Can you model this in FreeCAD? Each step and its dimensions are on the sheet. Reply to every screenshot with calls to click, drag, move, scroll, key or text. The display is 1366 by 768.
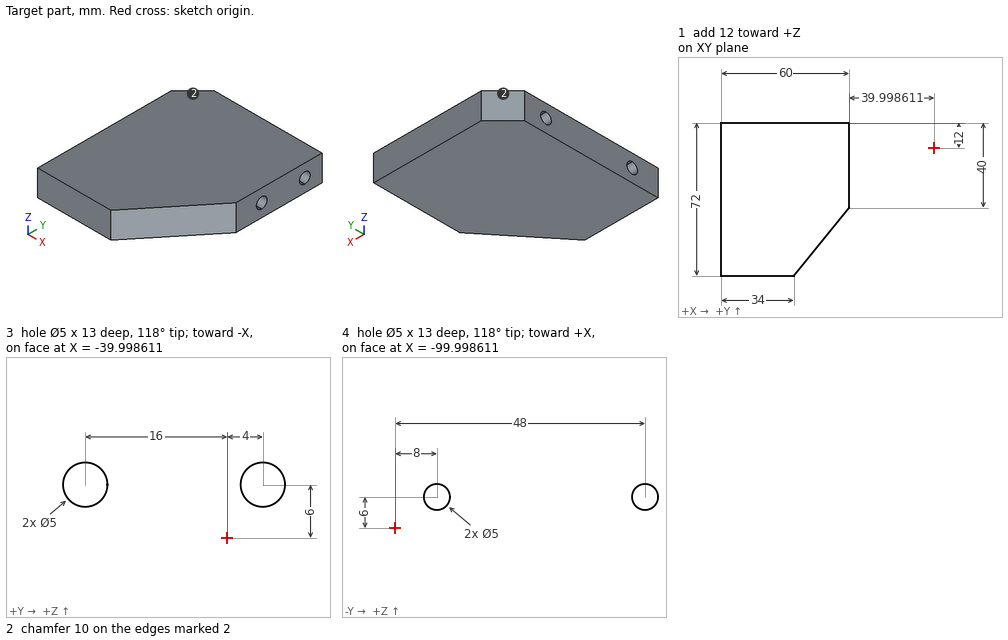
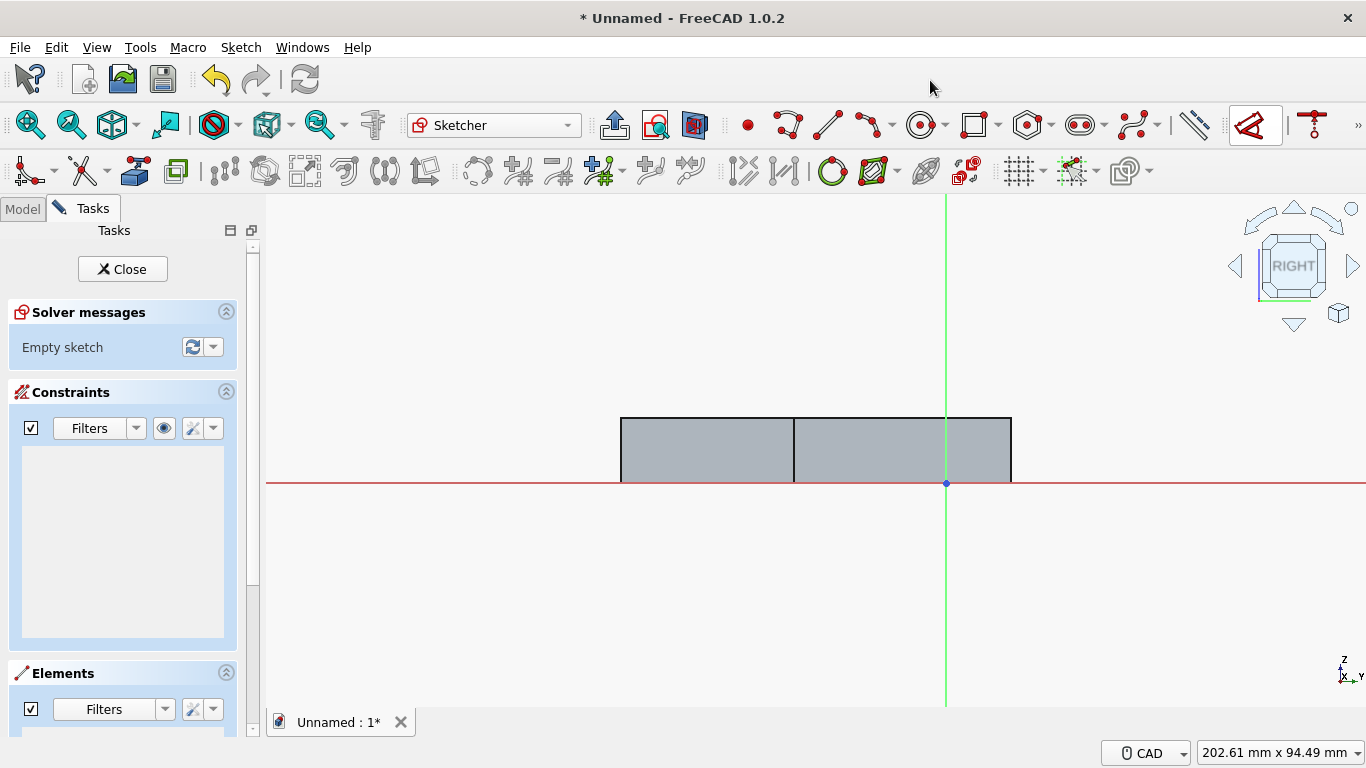
scroll(956, 462, up, 8)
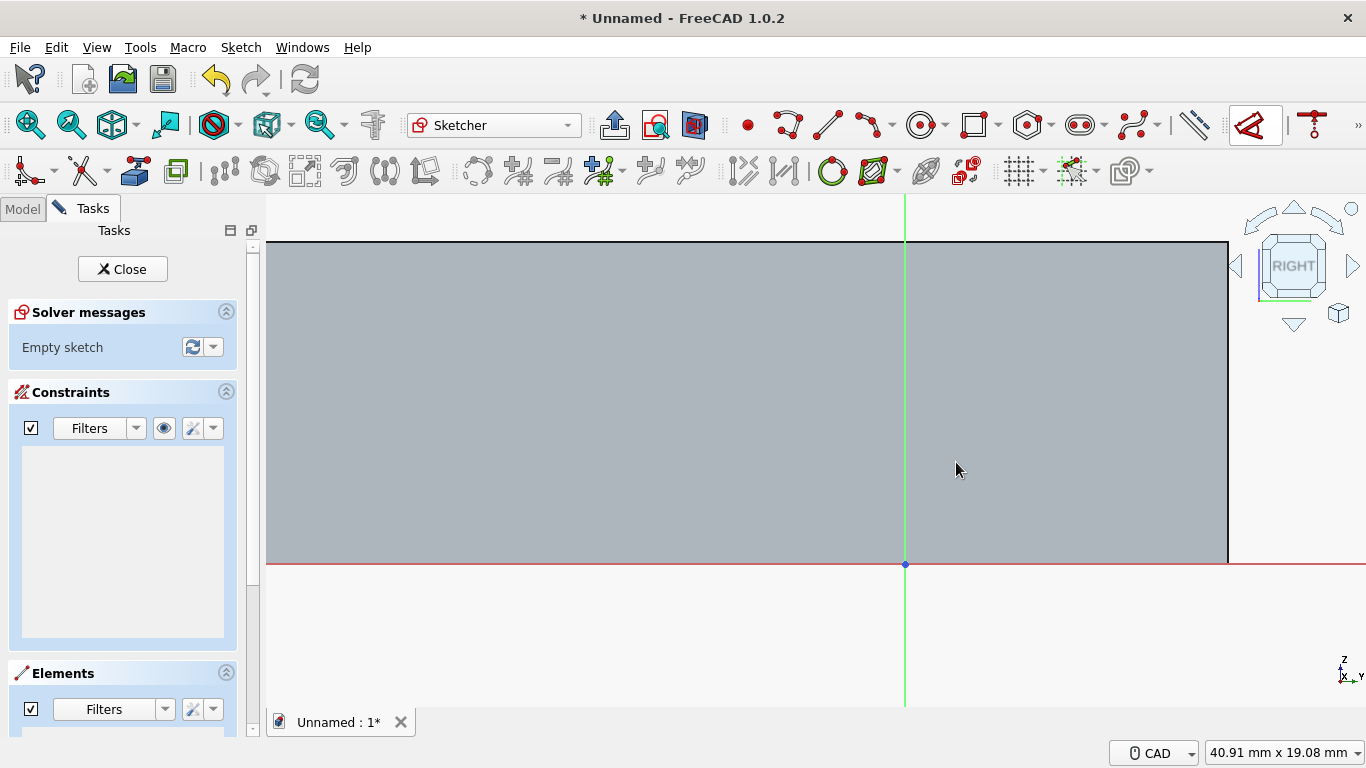
click(922, 126)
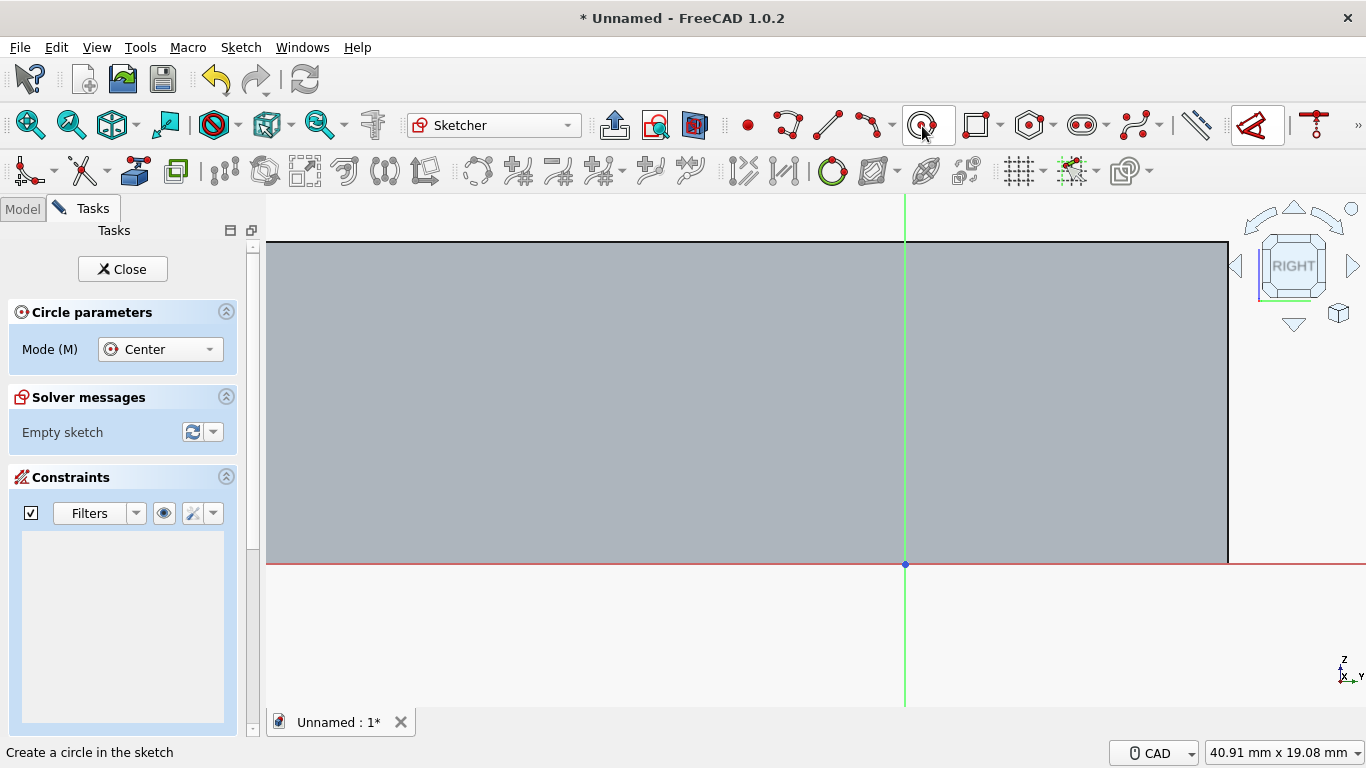
click(1013, 403)
move(1061, 355)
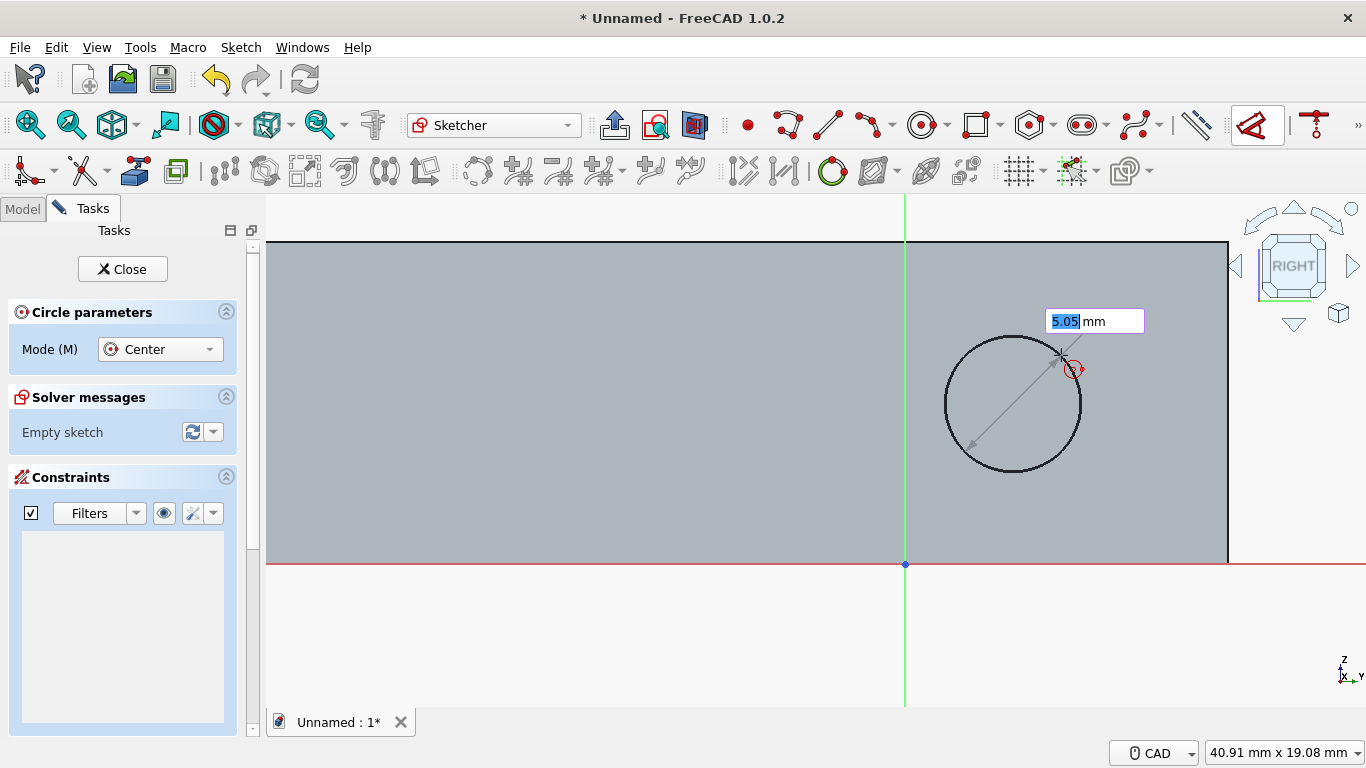
text(5)
key(Return)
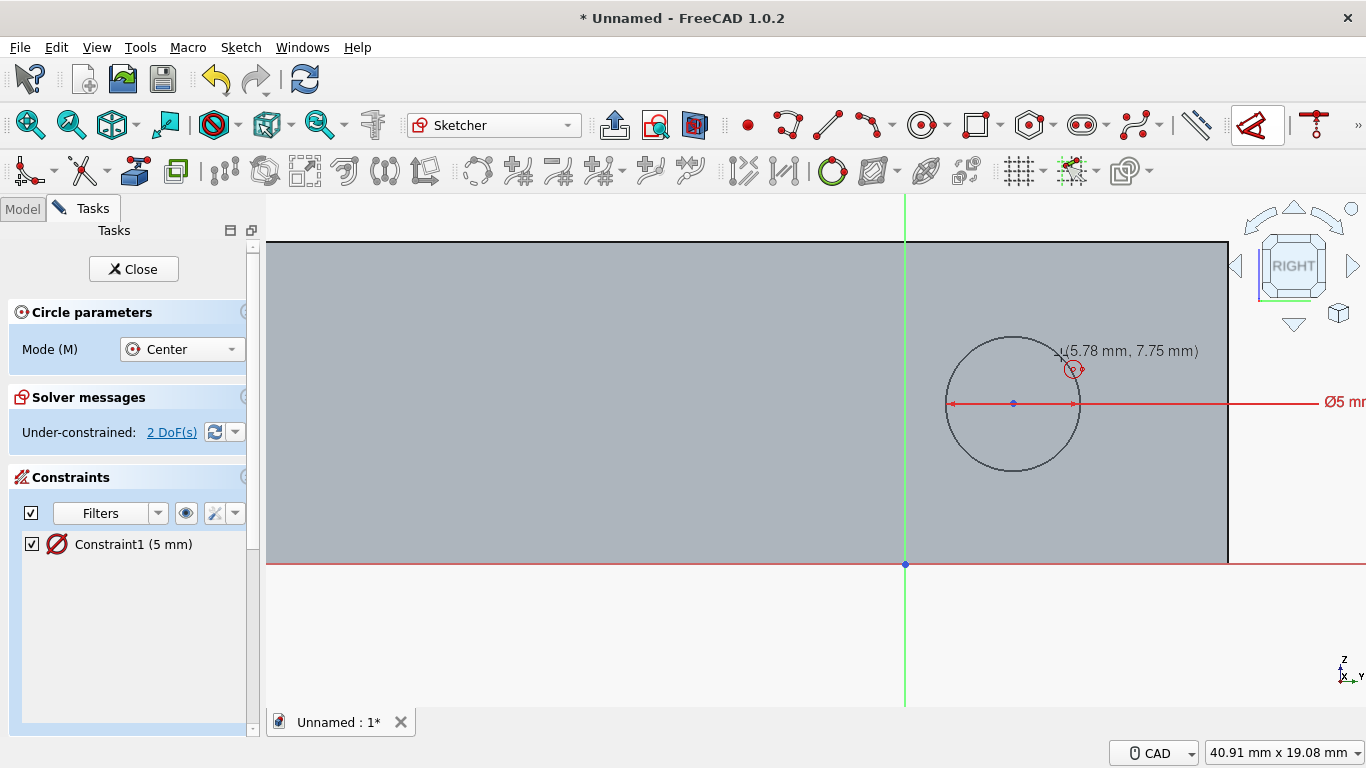
click(475, 403)
move(523, 355)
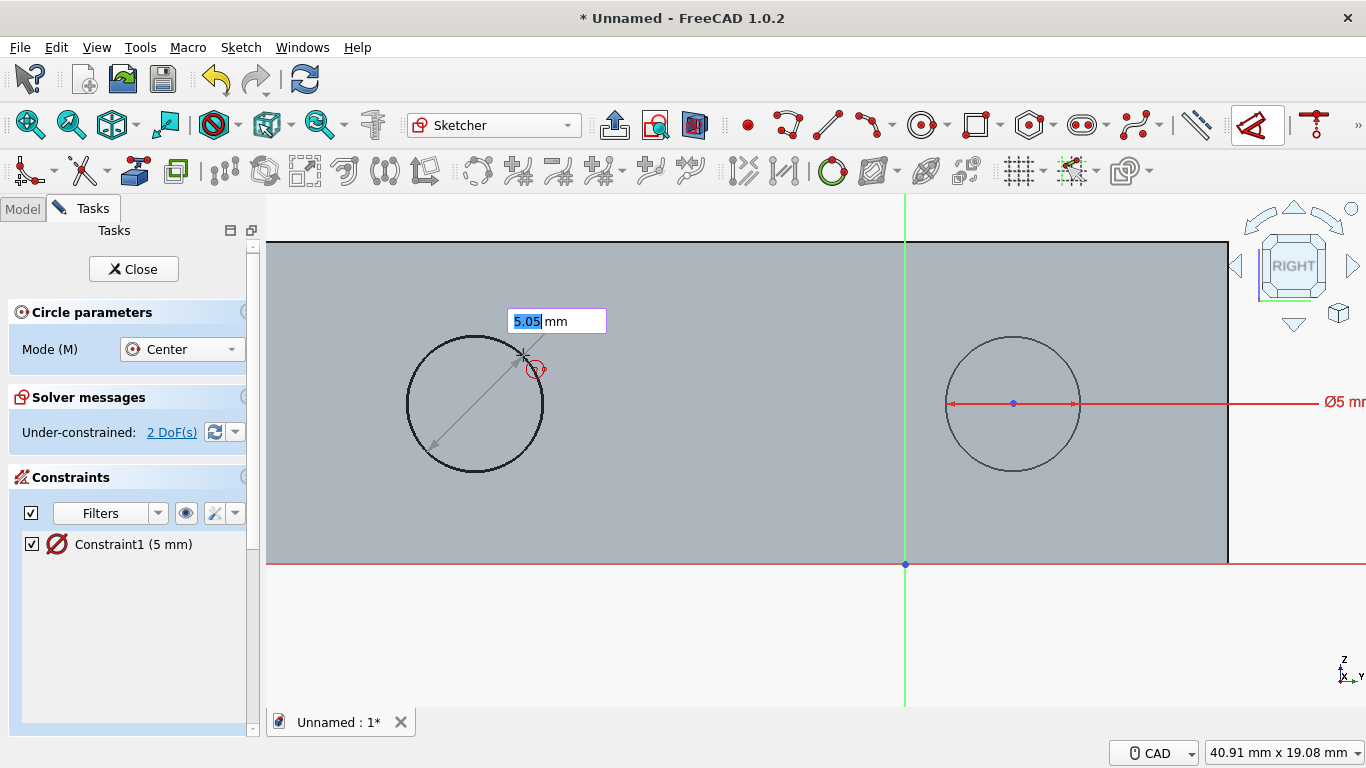
text(5)
key(Return)
key(Escape)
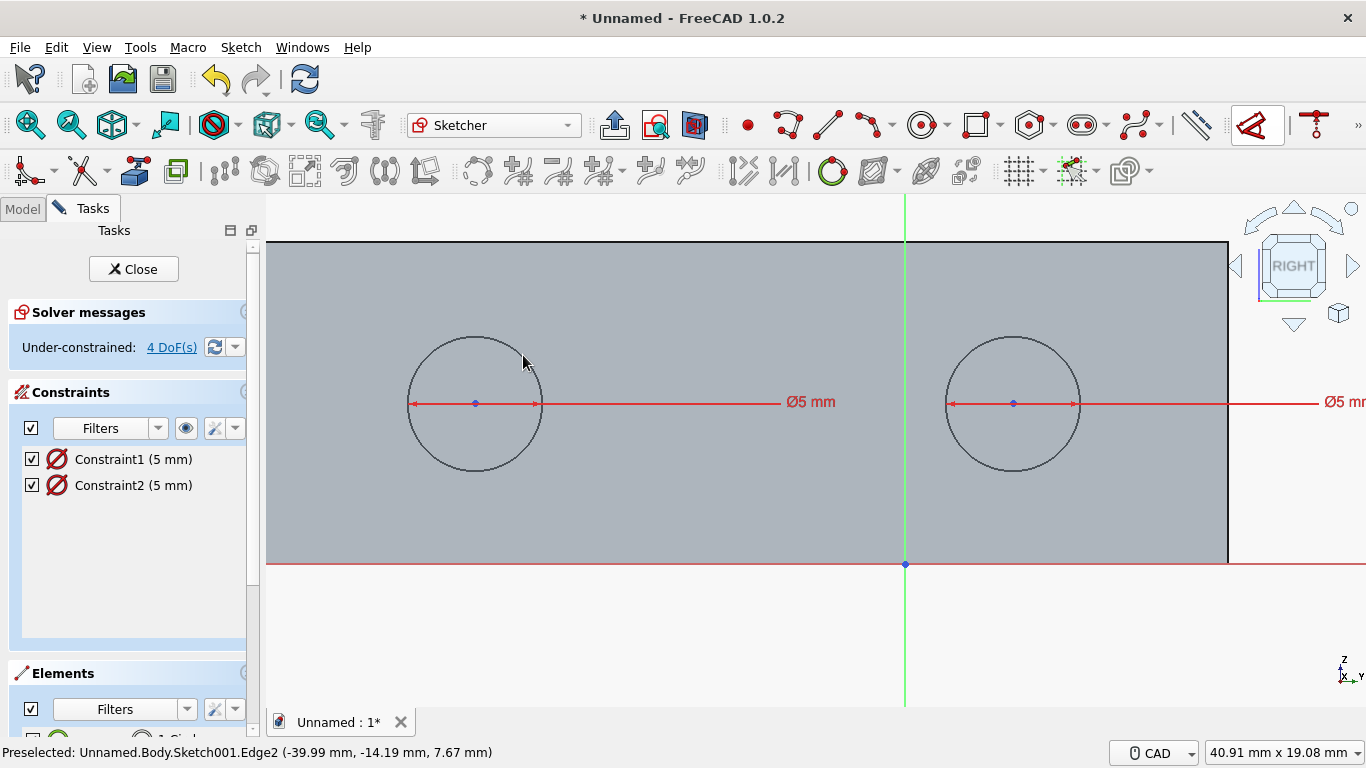
click(1013, 404)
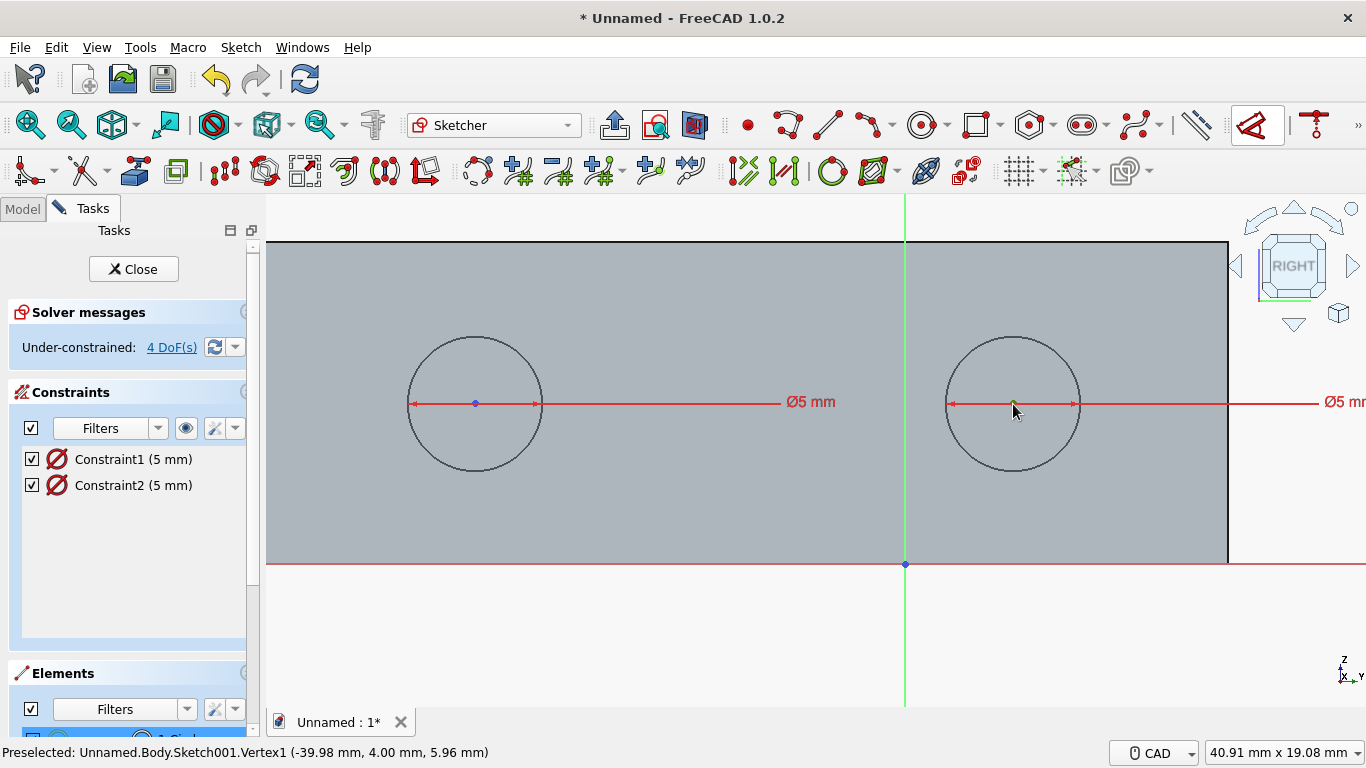
click(475, 404)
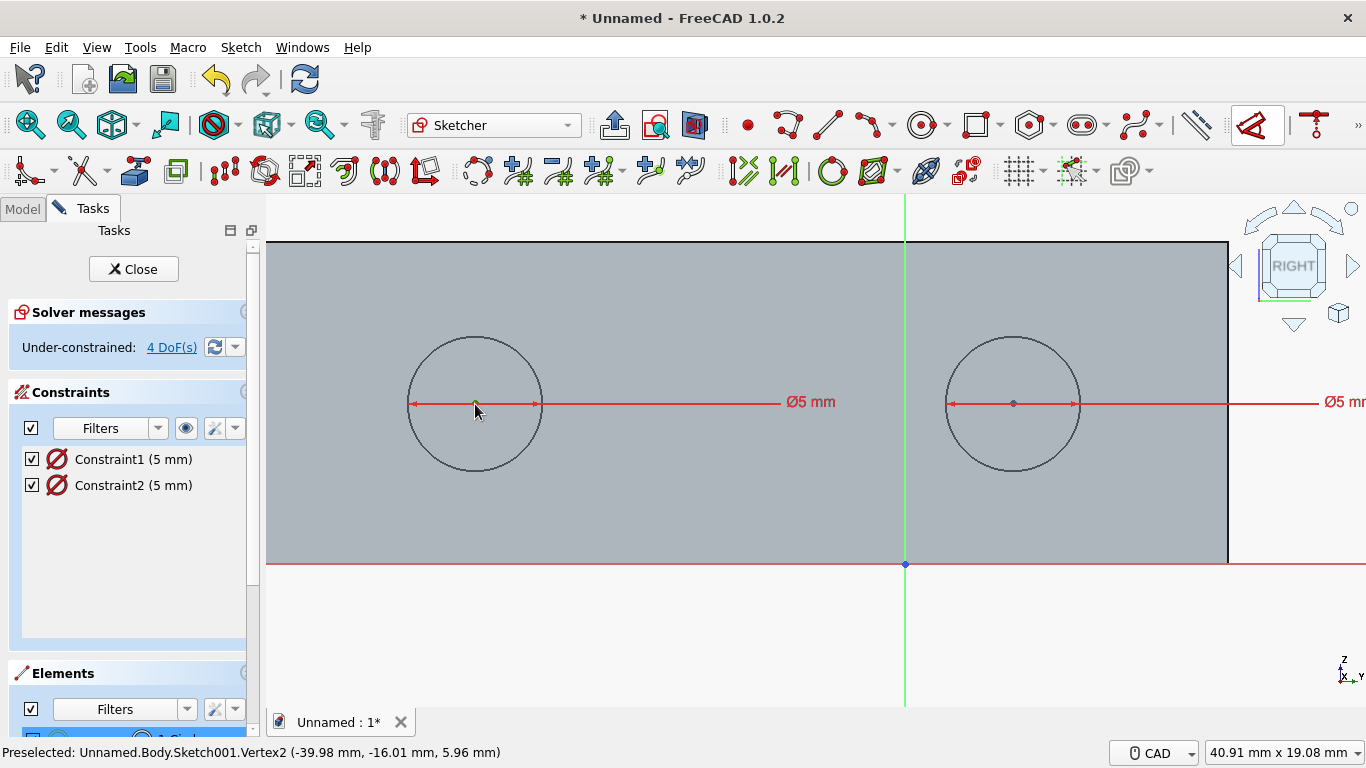
key(h)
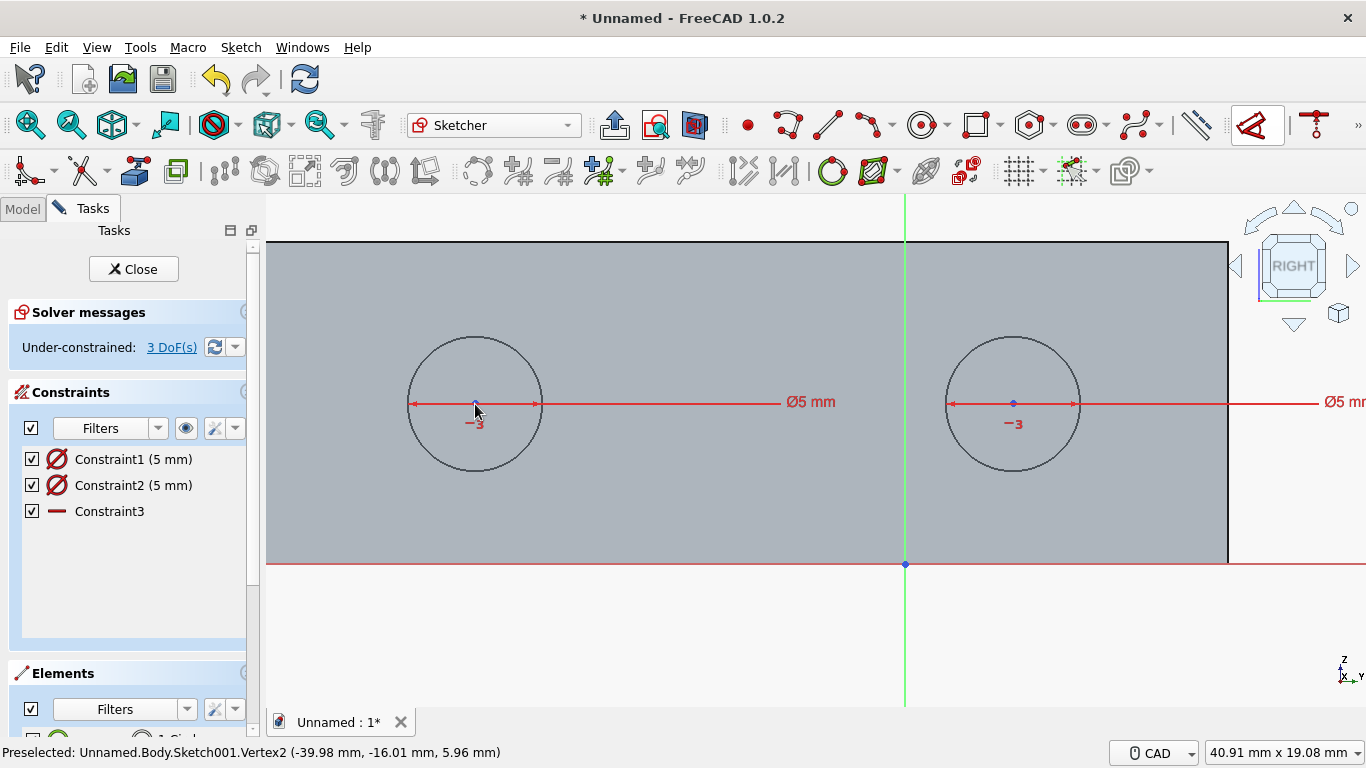
click(1013, 404)